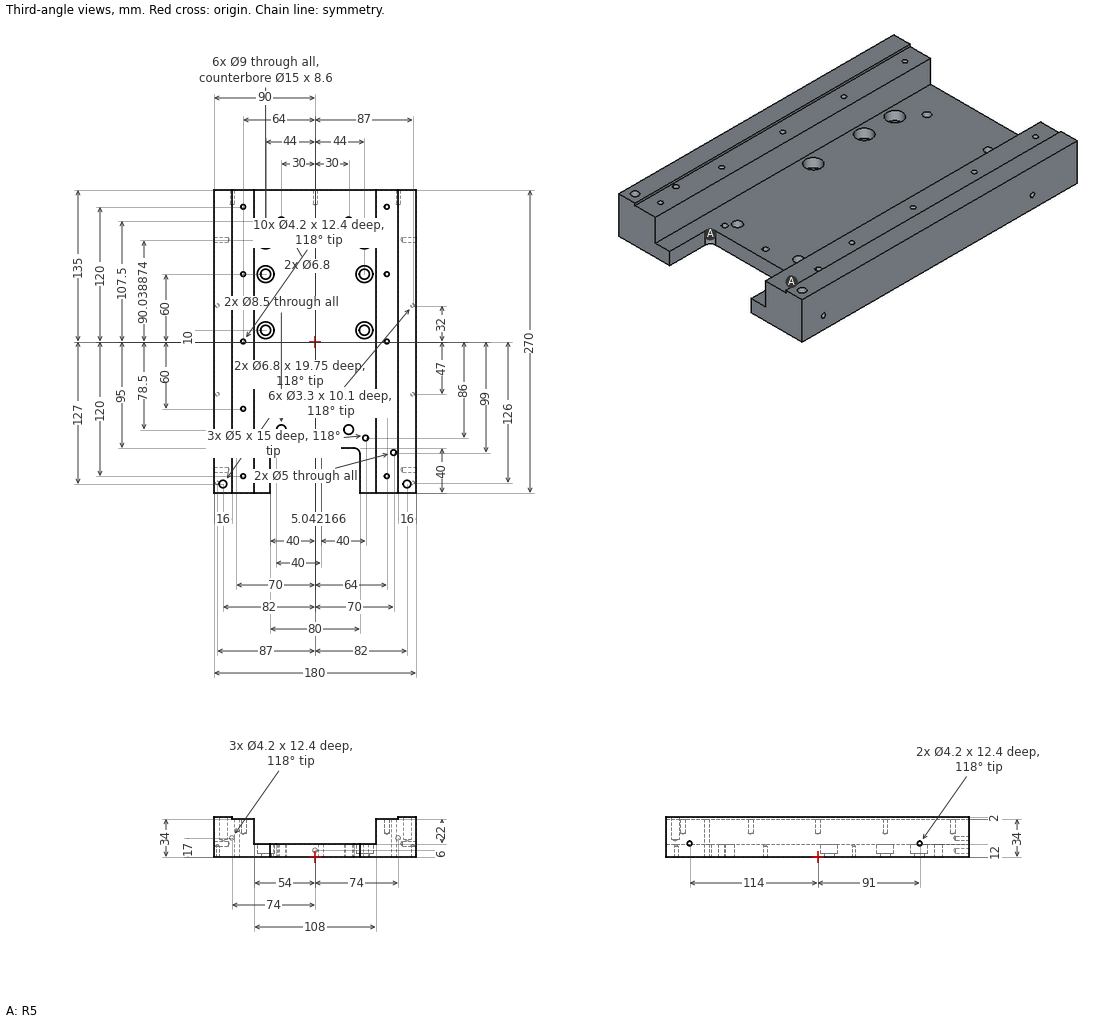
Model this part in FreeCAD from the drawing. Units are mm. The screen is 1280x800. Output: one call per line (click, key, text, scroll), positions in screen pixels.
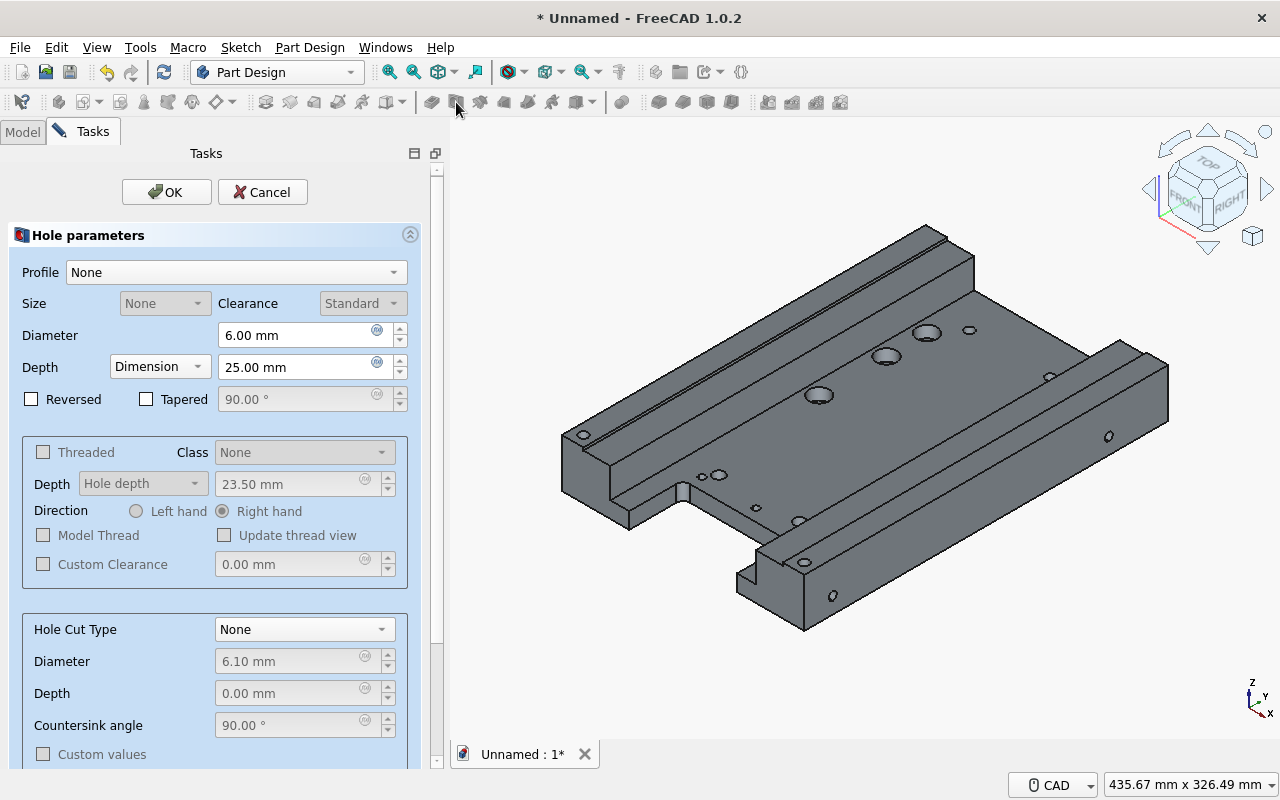
triple_click(305, 335)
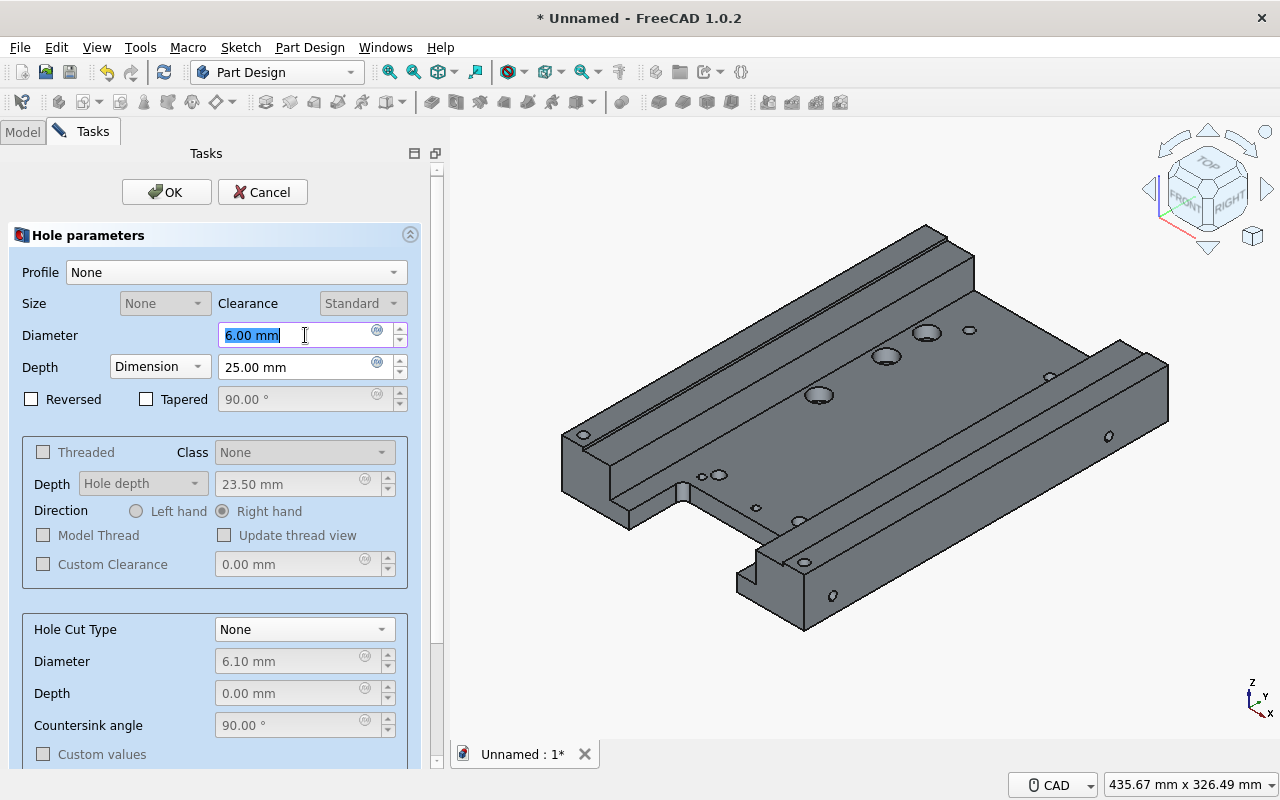
text(4.2)
key(Tab)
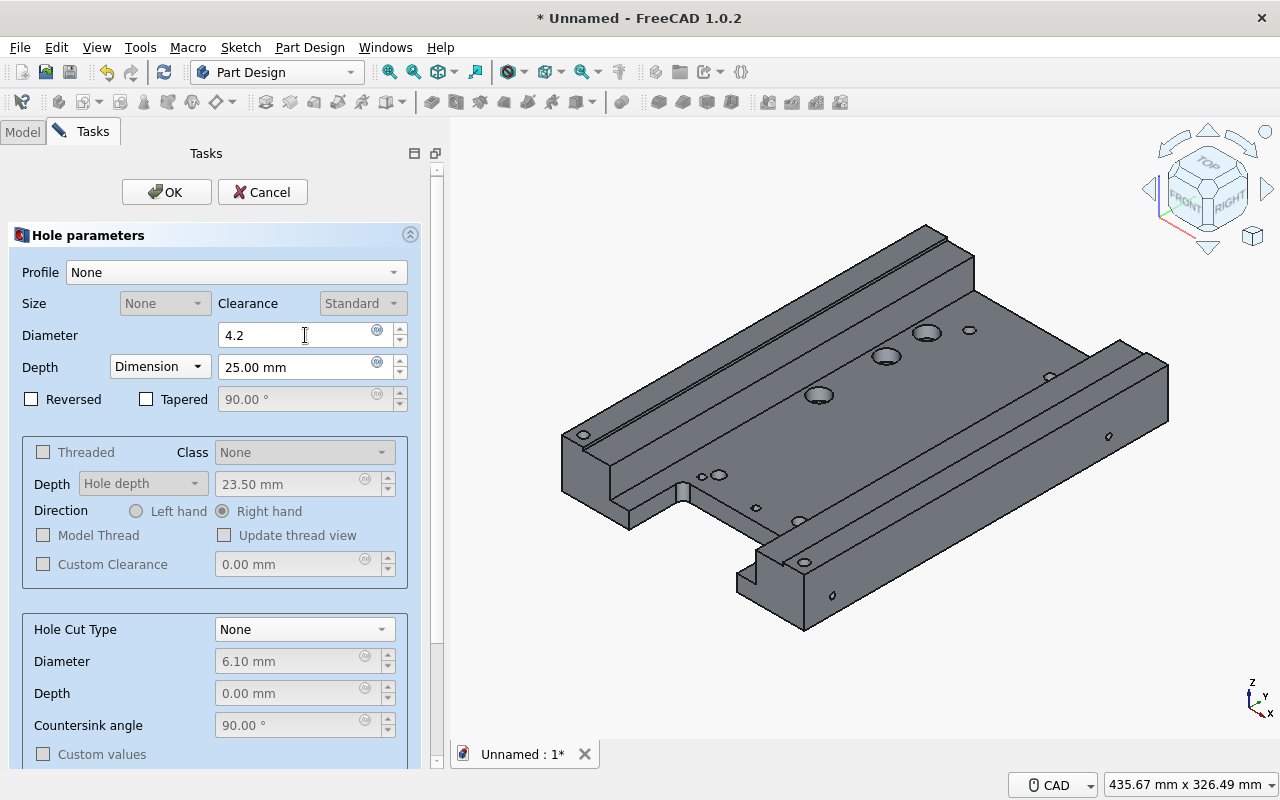
triple_click(305, 367)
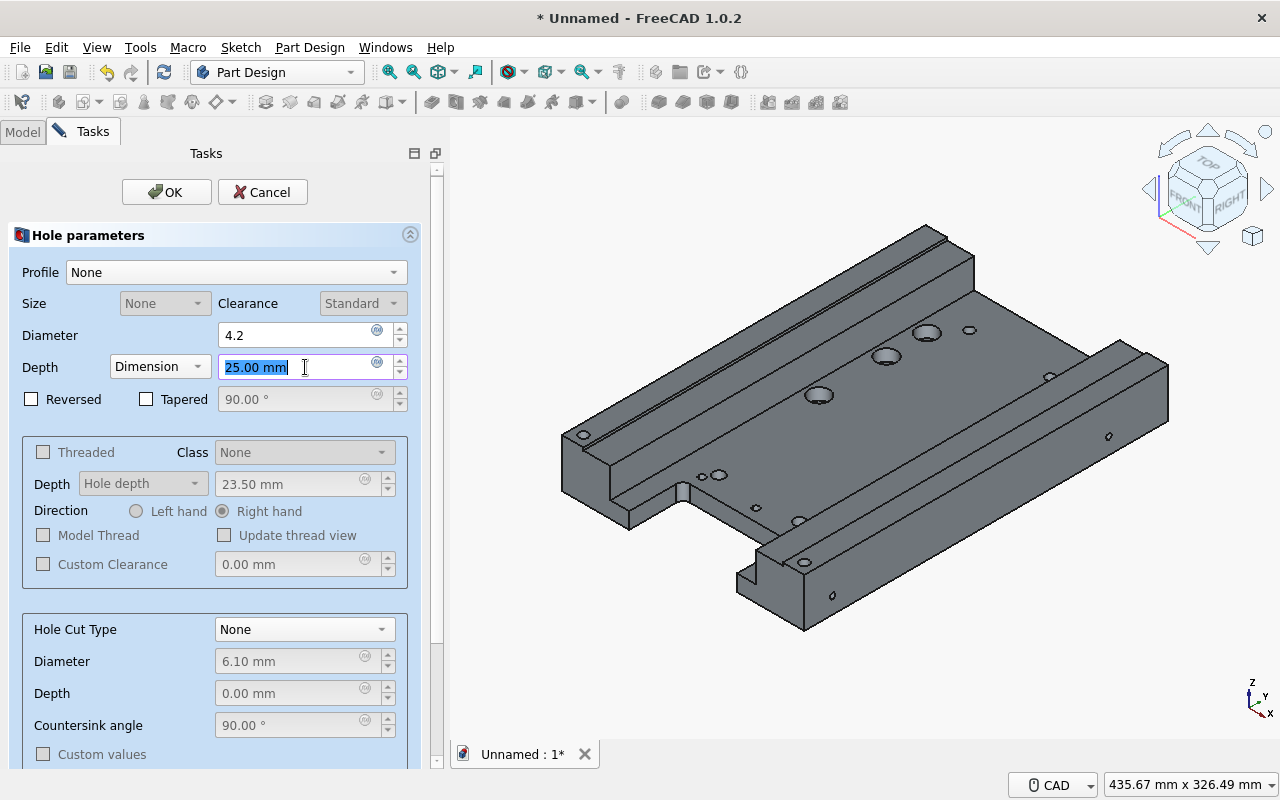
text(12.4)
key(Tab)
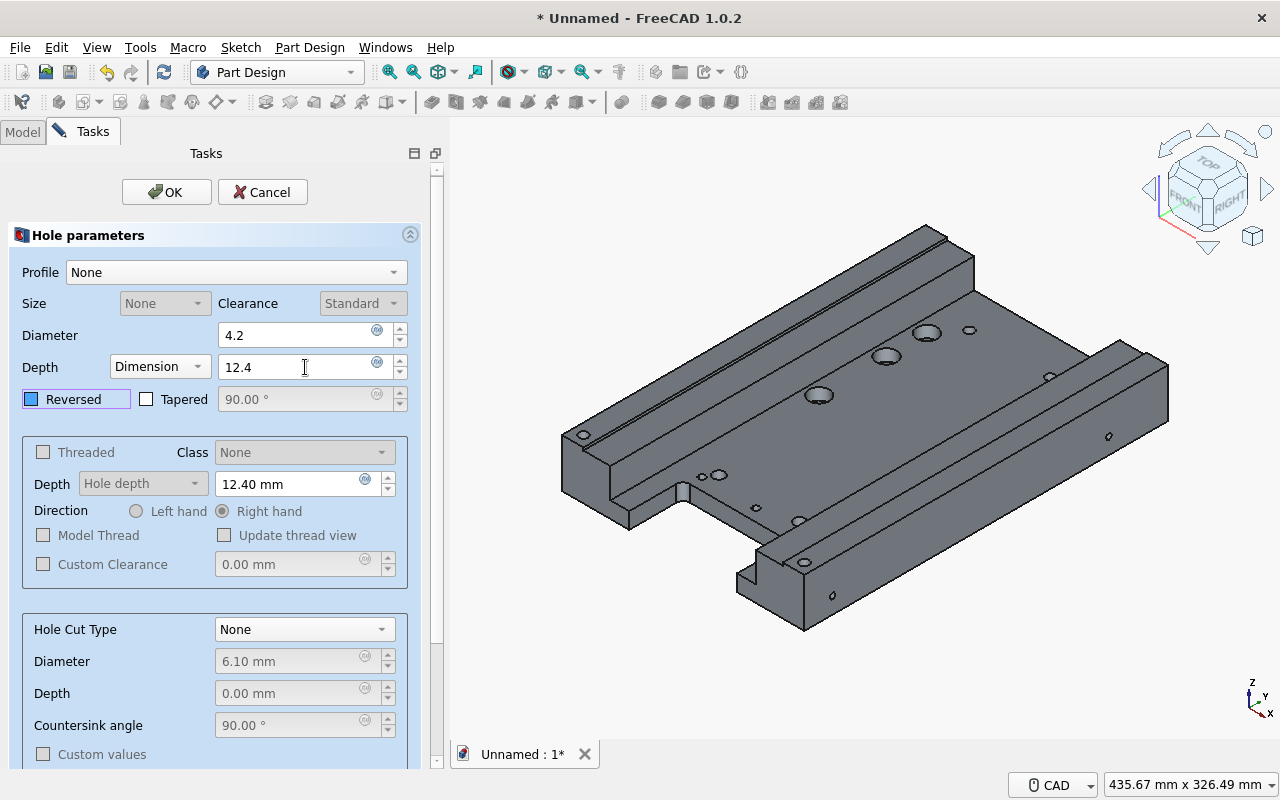
click(167, 192)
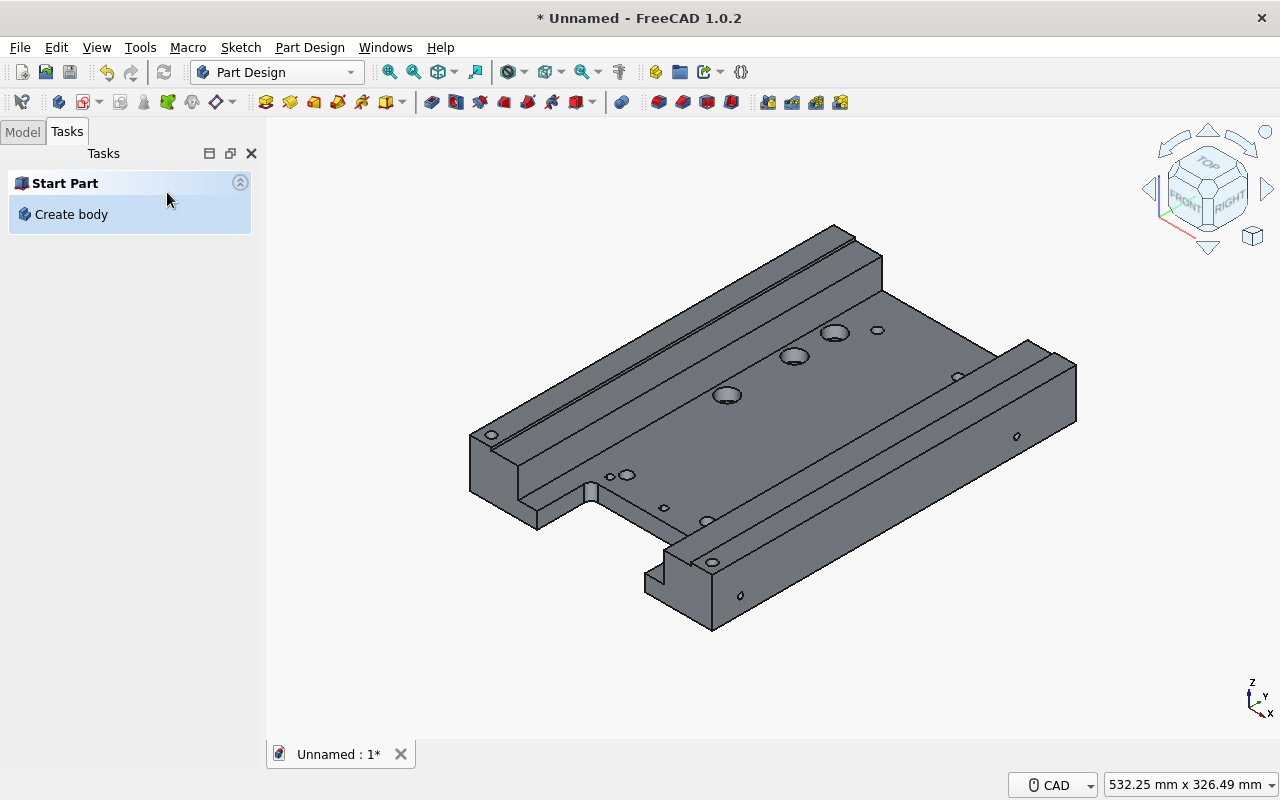
click(84, 102)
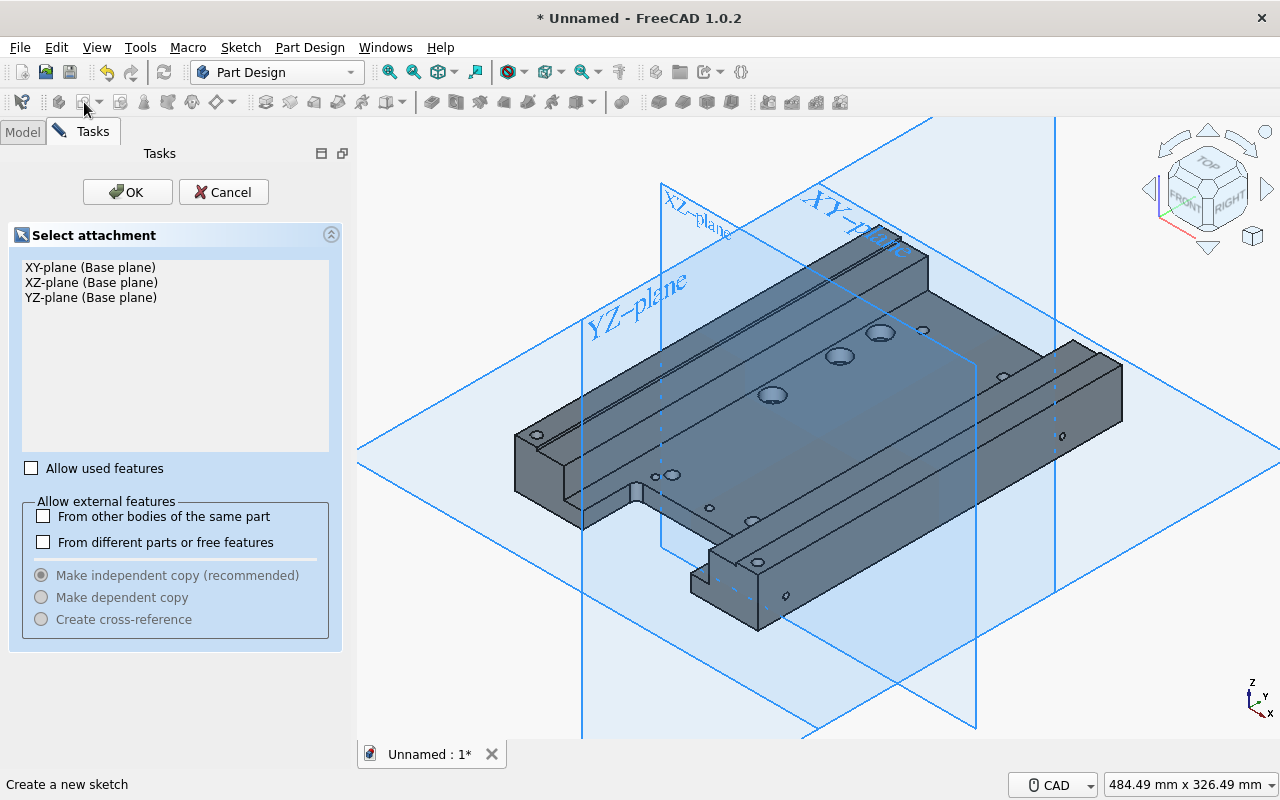
click(82, 268)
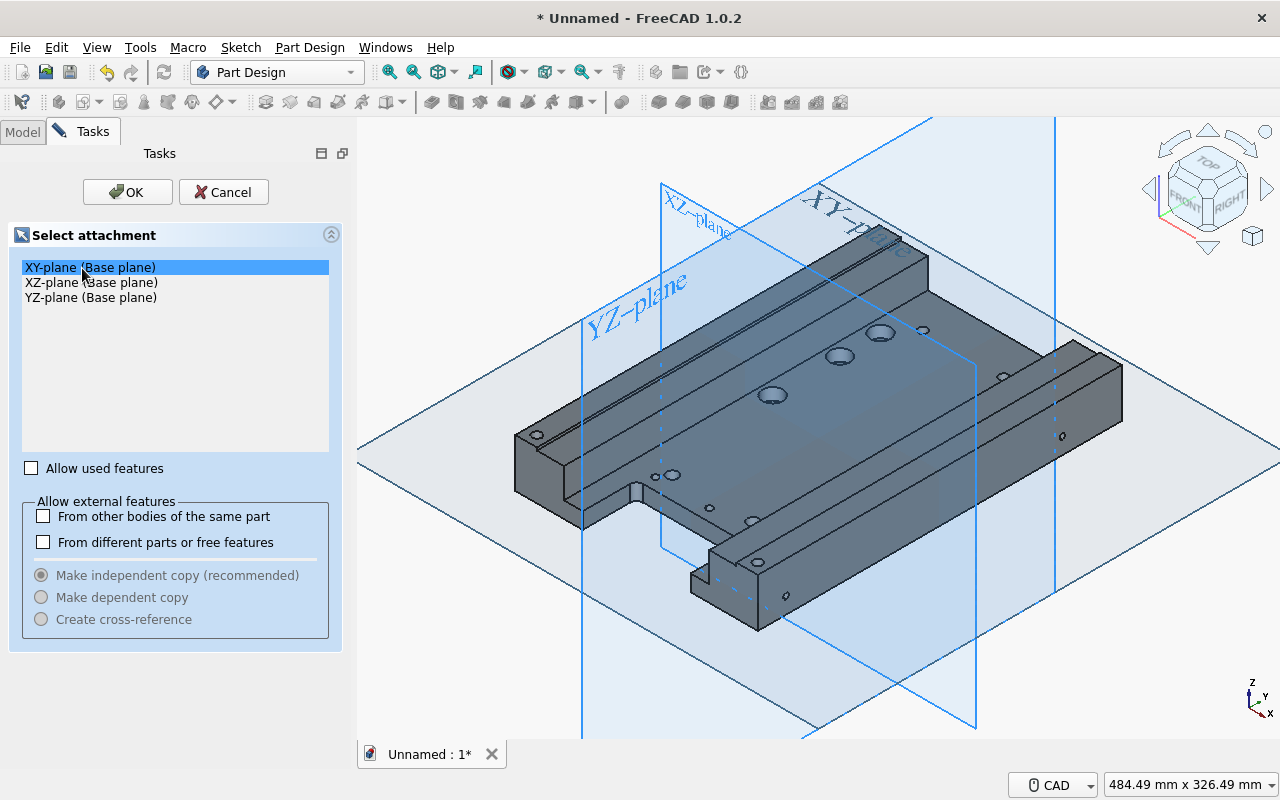
click(128, 192)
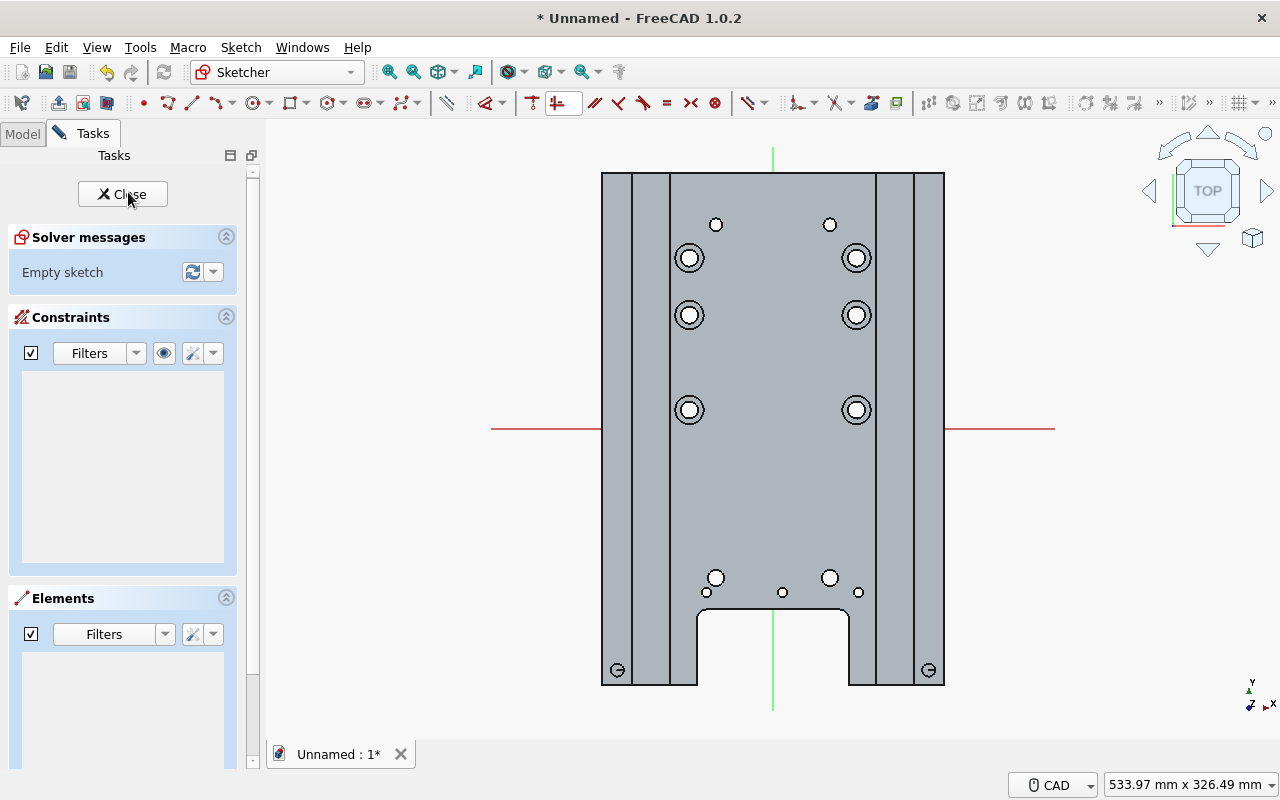
click(108, 104)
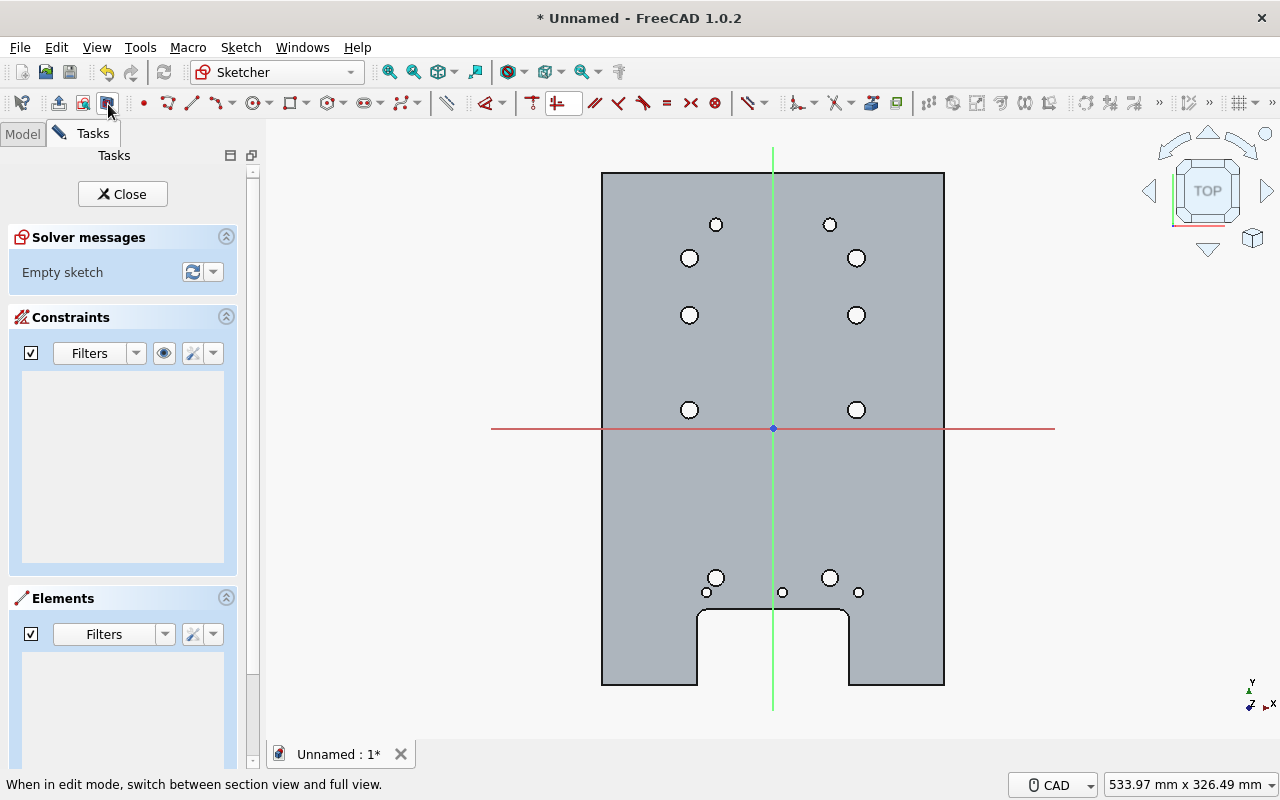
scroll(829, 604, up, 4)